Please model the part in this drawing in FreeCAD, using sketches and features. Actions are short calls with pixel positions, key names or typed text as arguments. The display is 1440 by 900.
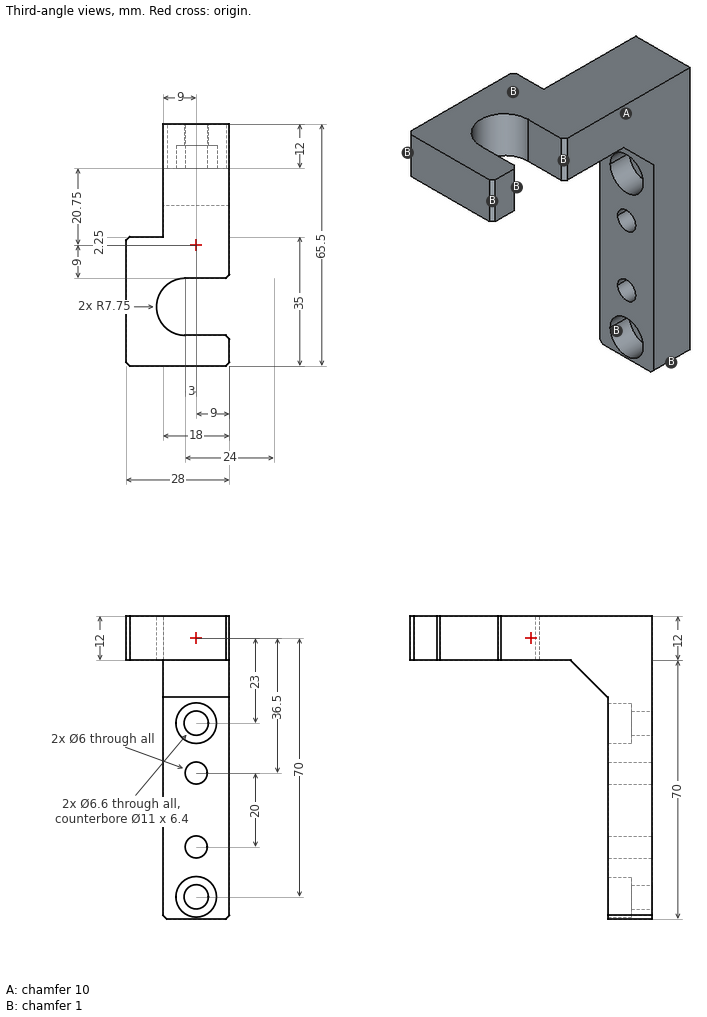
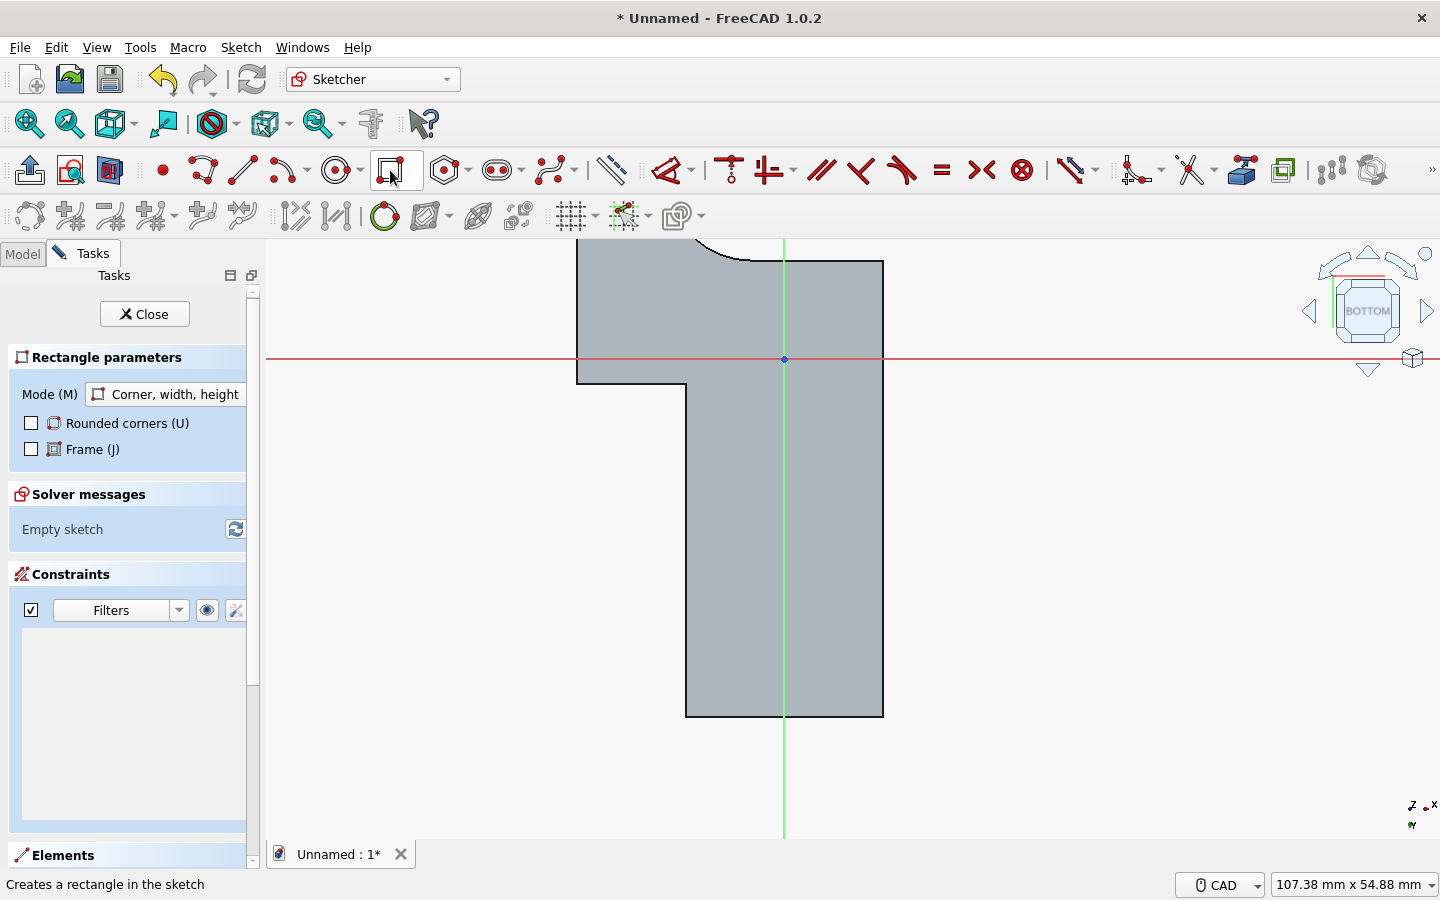
click(686, 586)
move(883, 717)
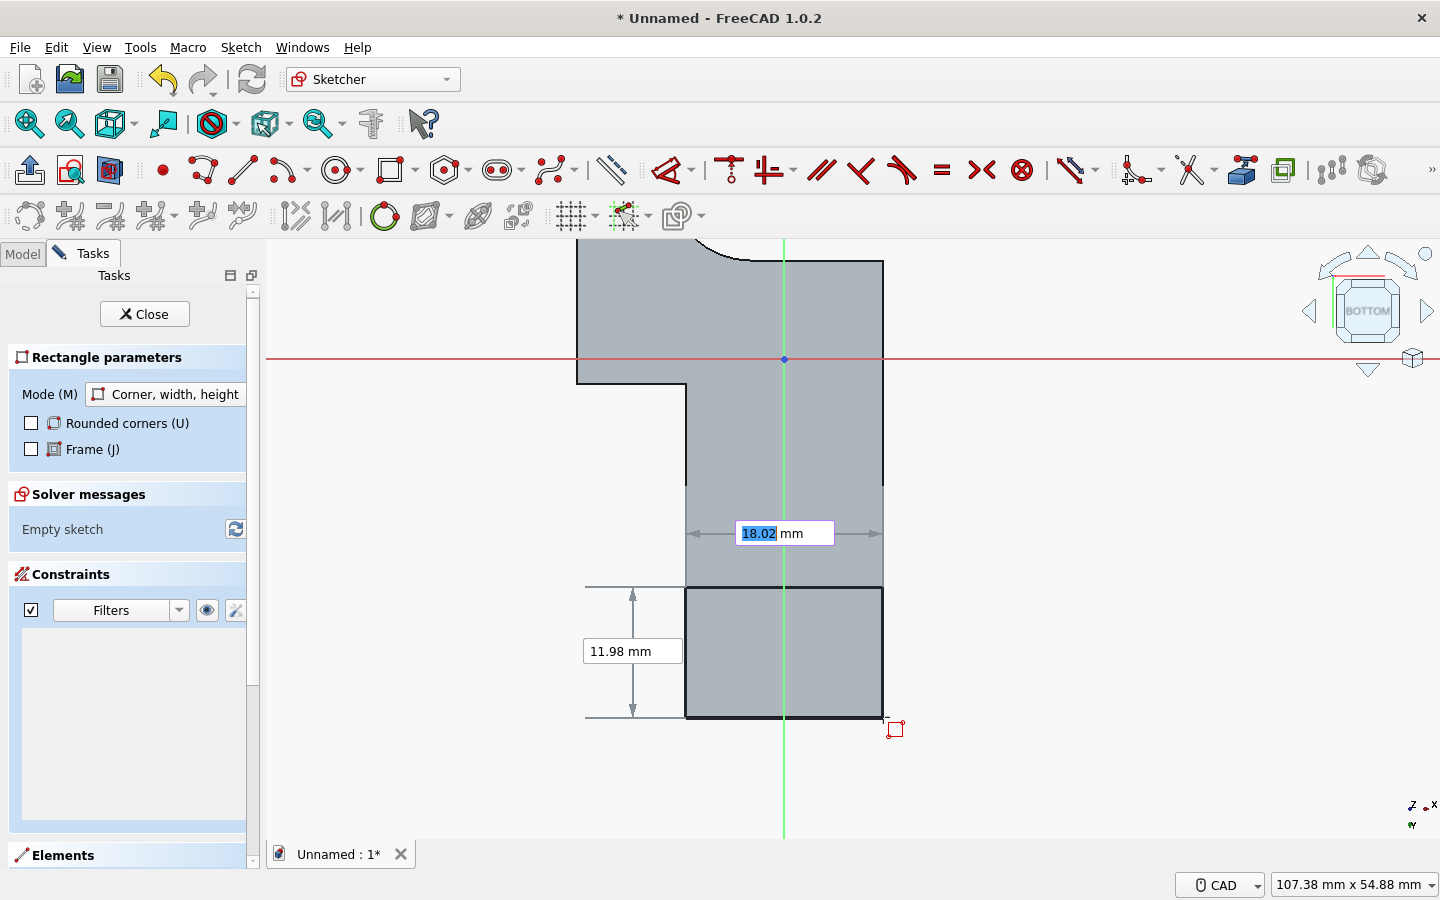
text(18)
key(Tab)
text(12)
key(Return)
key(Escape)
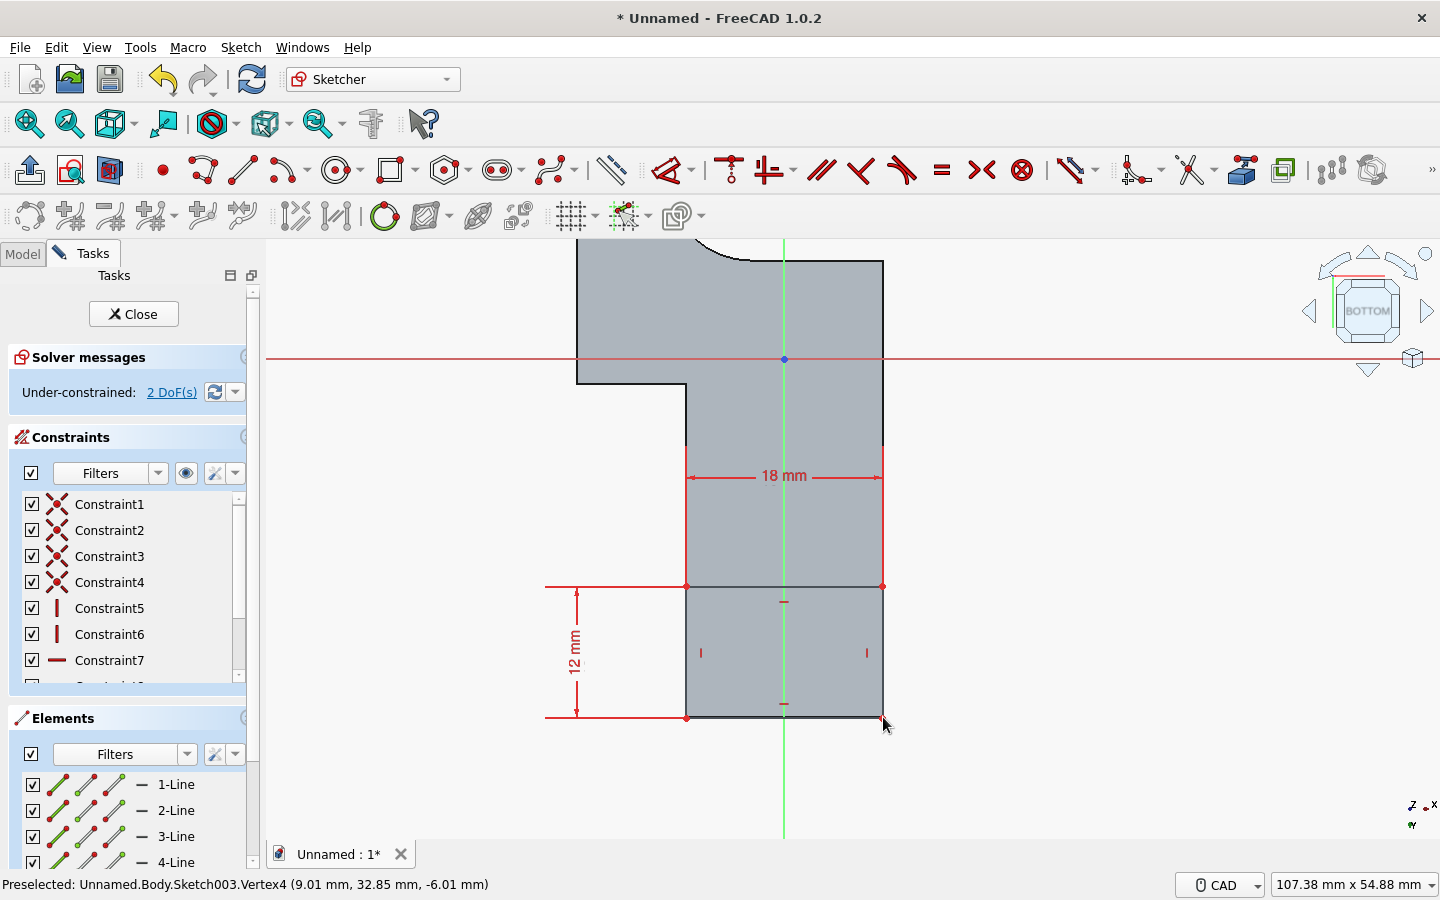
key(d)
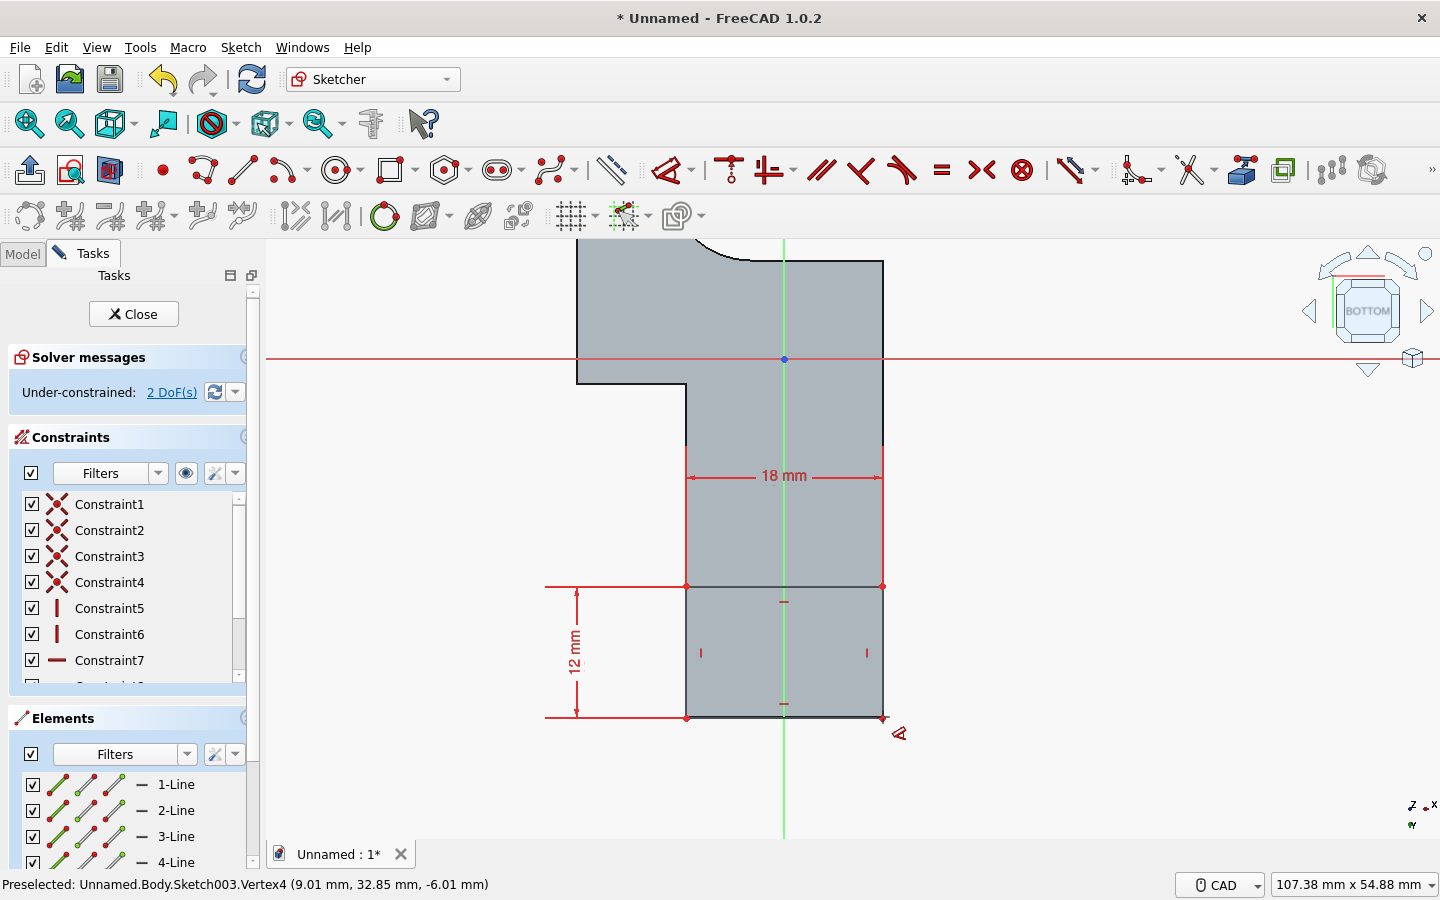
click(686, 587)
click(735, 325)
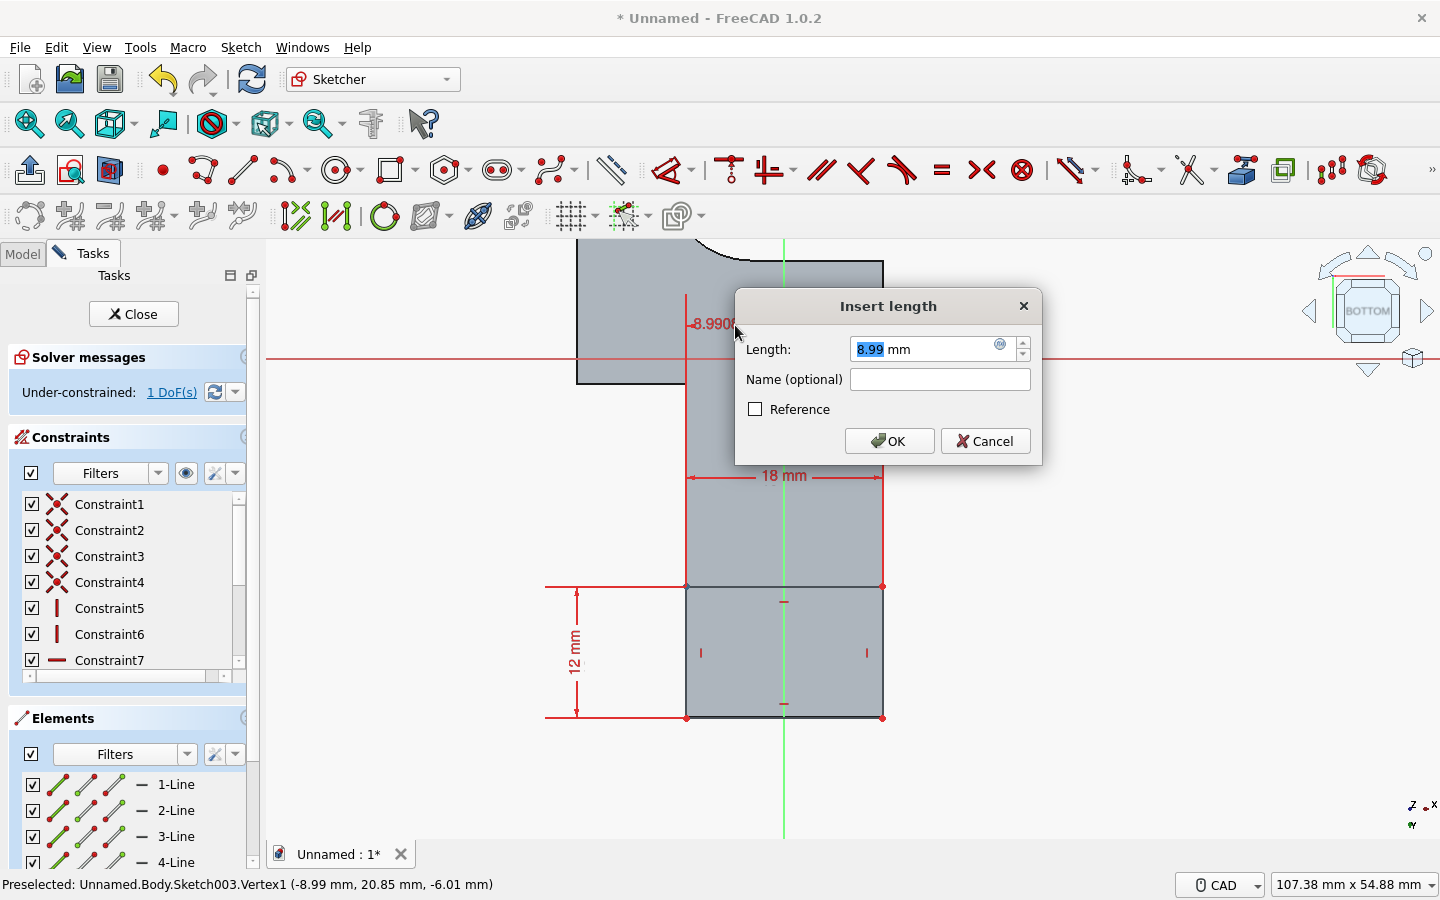
text(9)
key(Return)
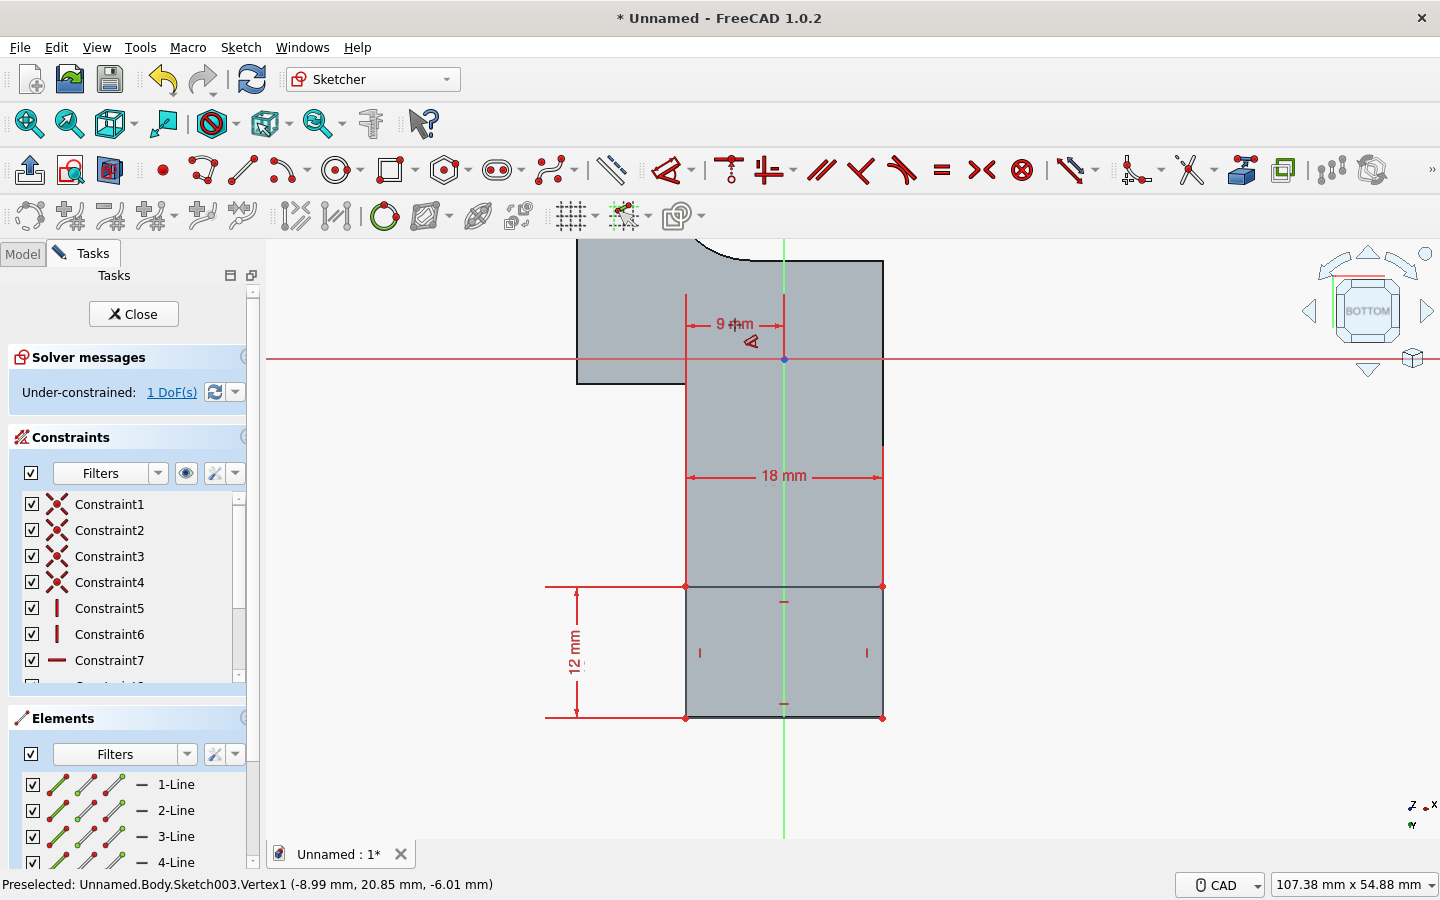
click(686, 587)
click(652, 473)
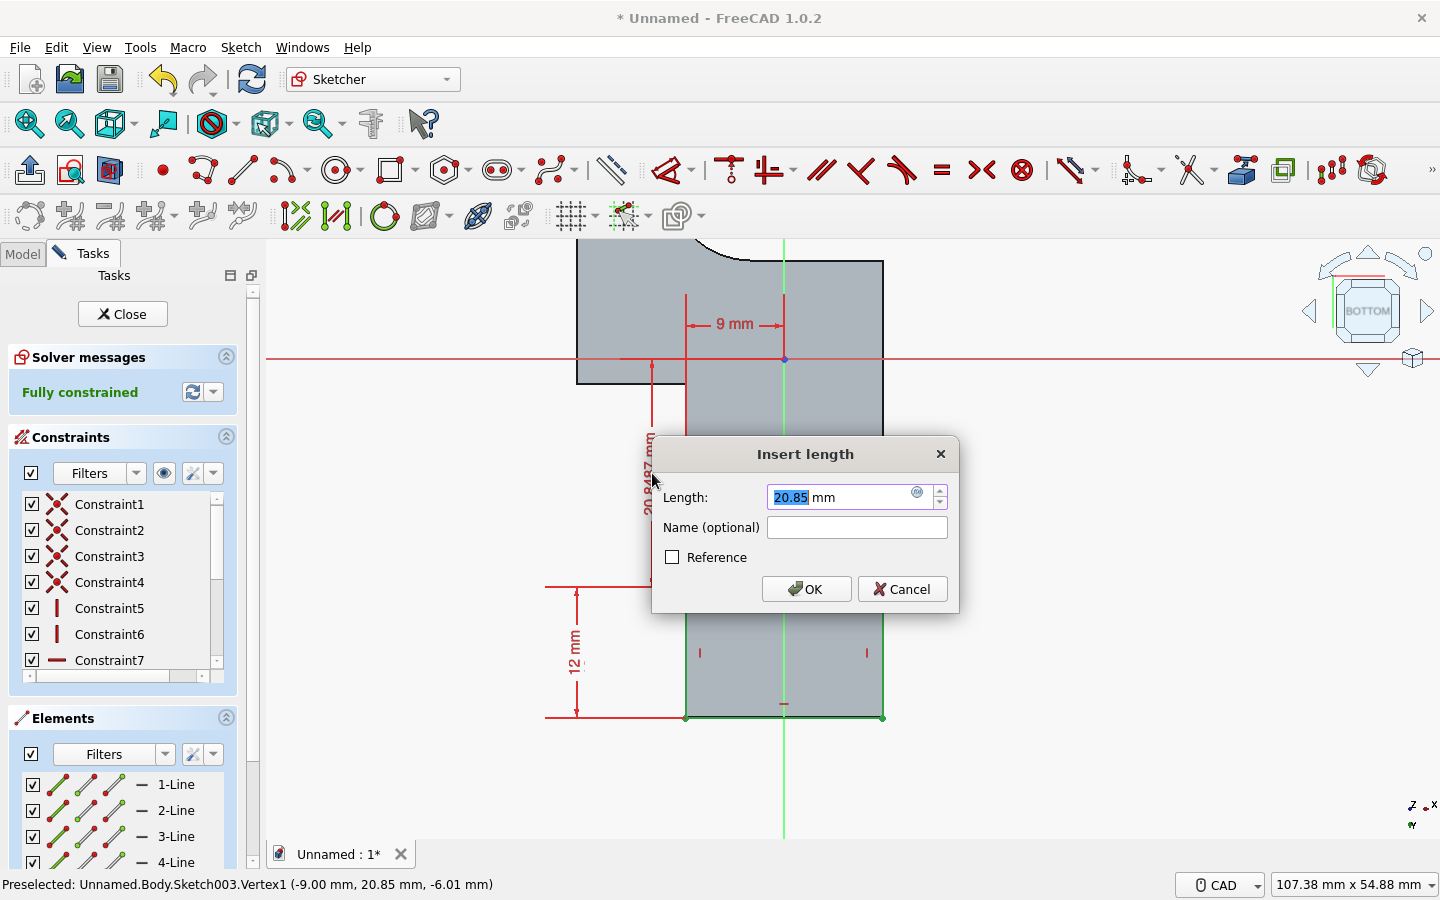
text(20.75)
key(Return)
key(Escape)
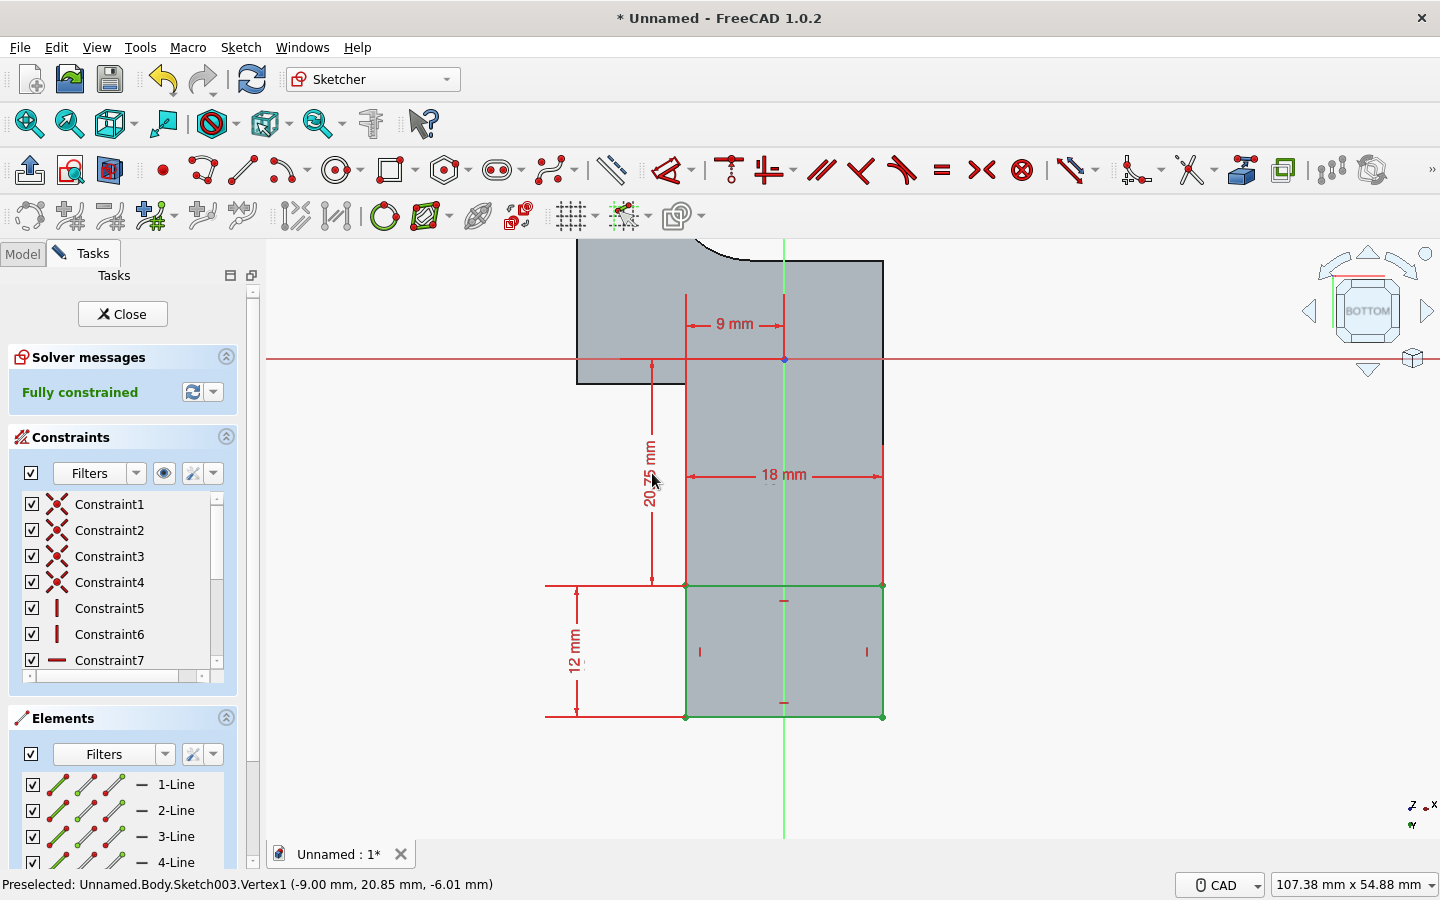
click(123, 314)